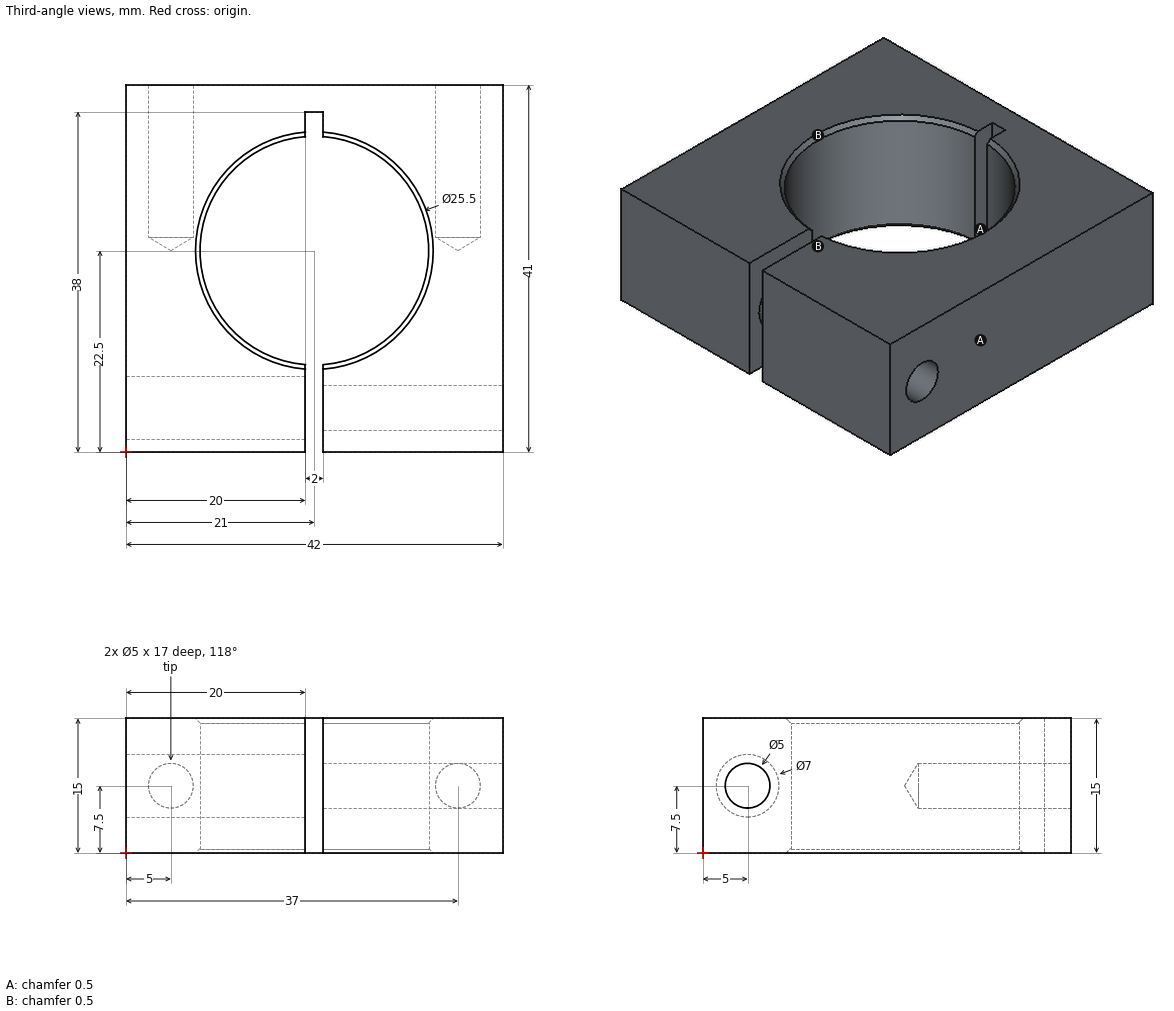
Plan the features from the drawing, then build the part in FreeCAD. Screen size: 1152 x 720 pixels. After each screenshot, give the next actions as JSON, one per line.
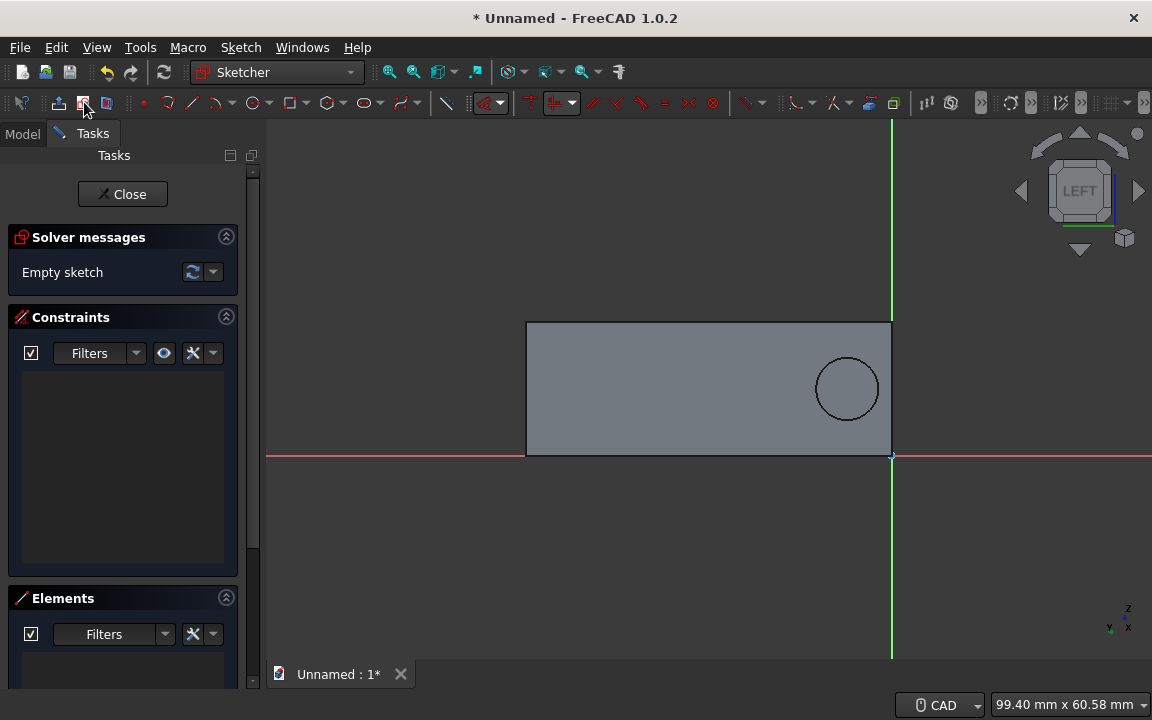
{"action": "scroll", "coordinate": [930, 419], "scroll_direction": "up", "scroll_amount": 7}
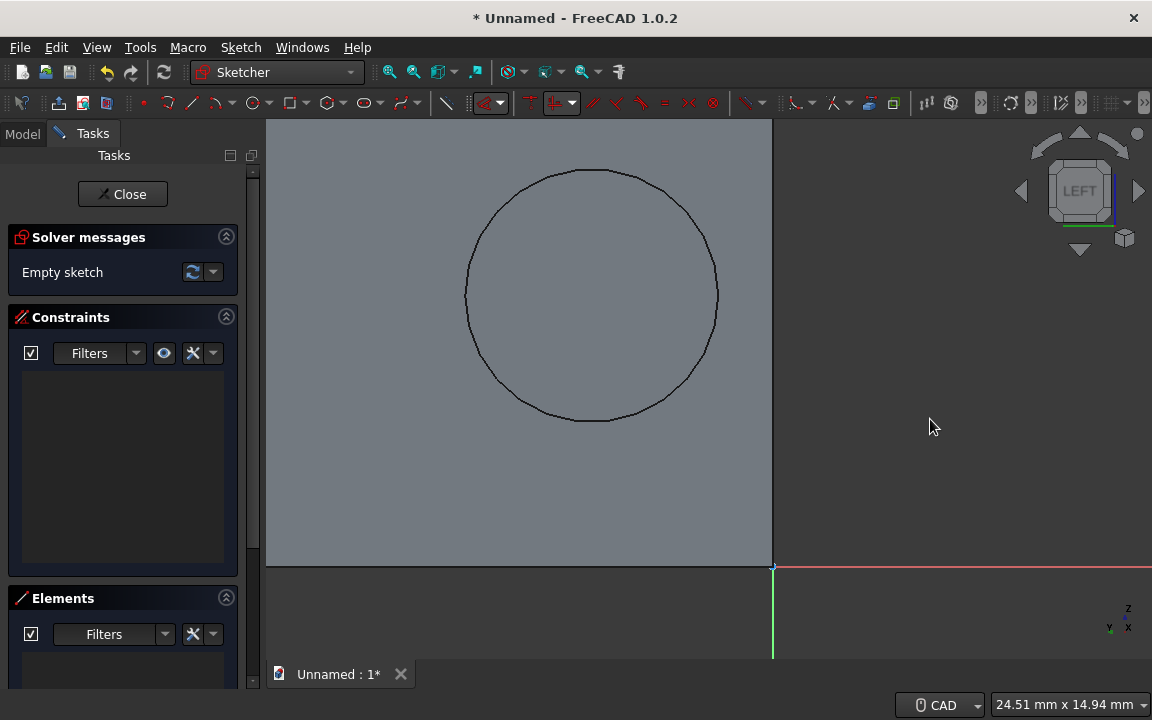
{"action": "left_click", "coordinate": [254, 104]}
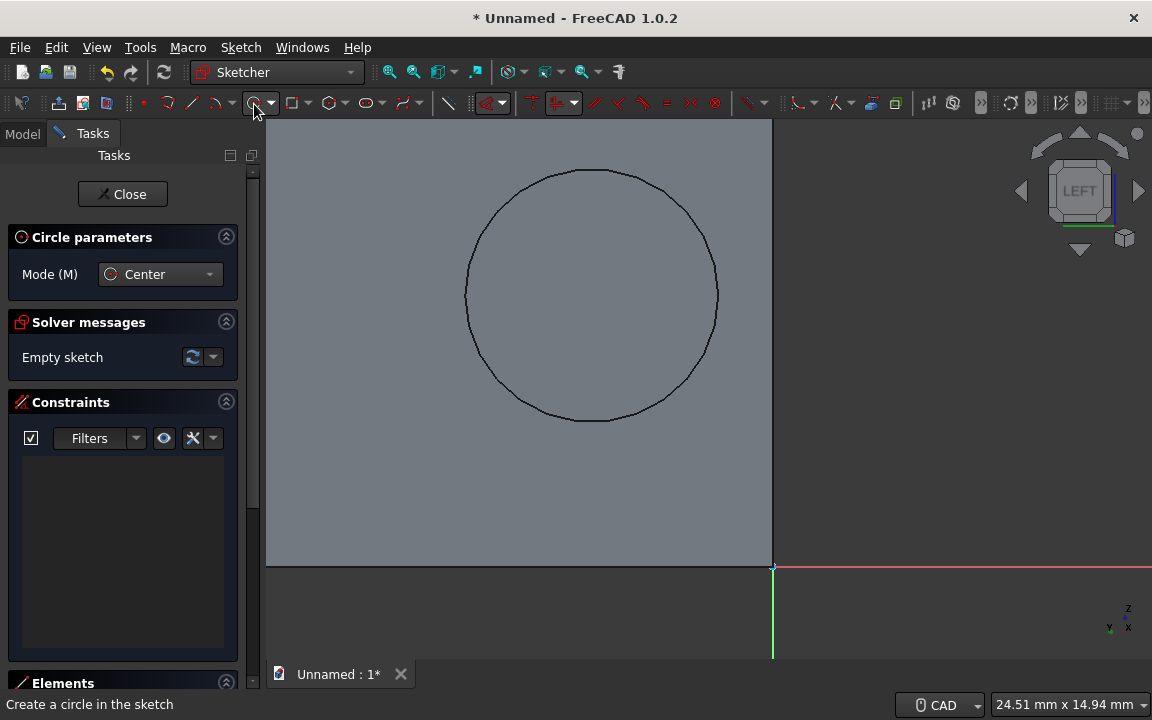
{"action": "left_click", "coordinate": [592, 296]}
{"action": "mouse_move", "coordinate": [656, 232]}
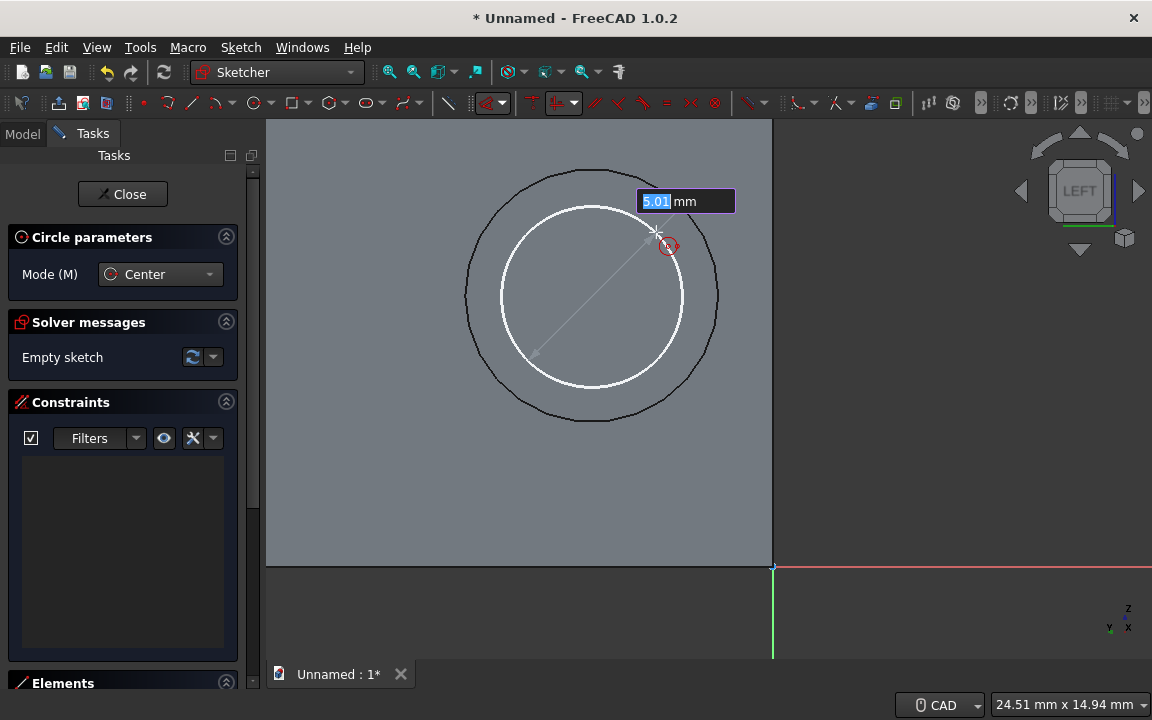
{"action": "type", "text": "5"}
{"action": "key", "text": "Return"}
{"action": "key", "text": "Escape"}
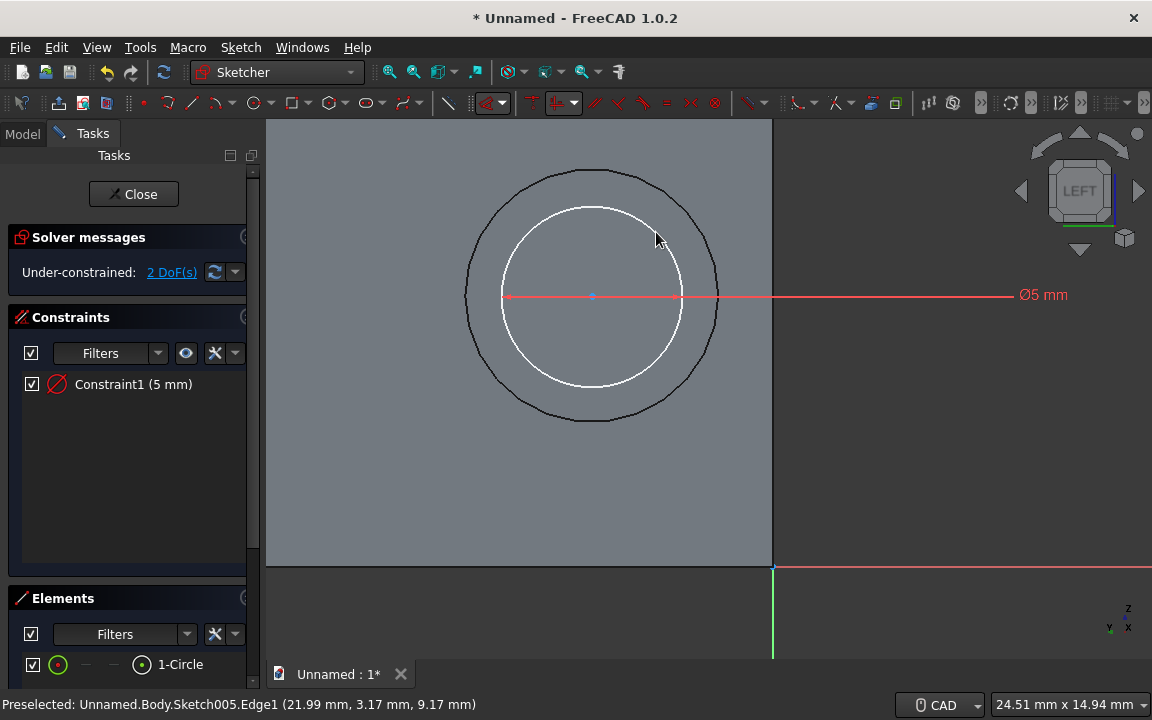
{"action": "left_click", "coordinate": [592, 297]}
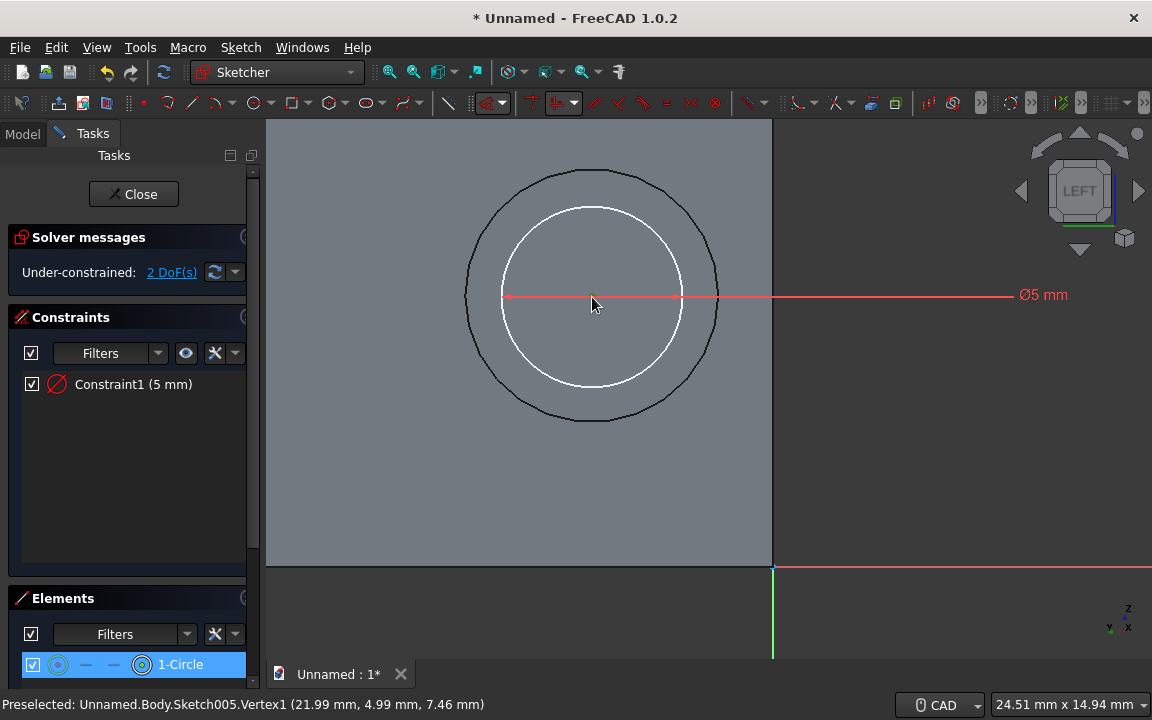
{"action": "left_click", "coordinate": [504, 104]}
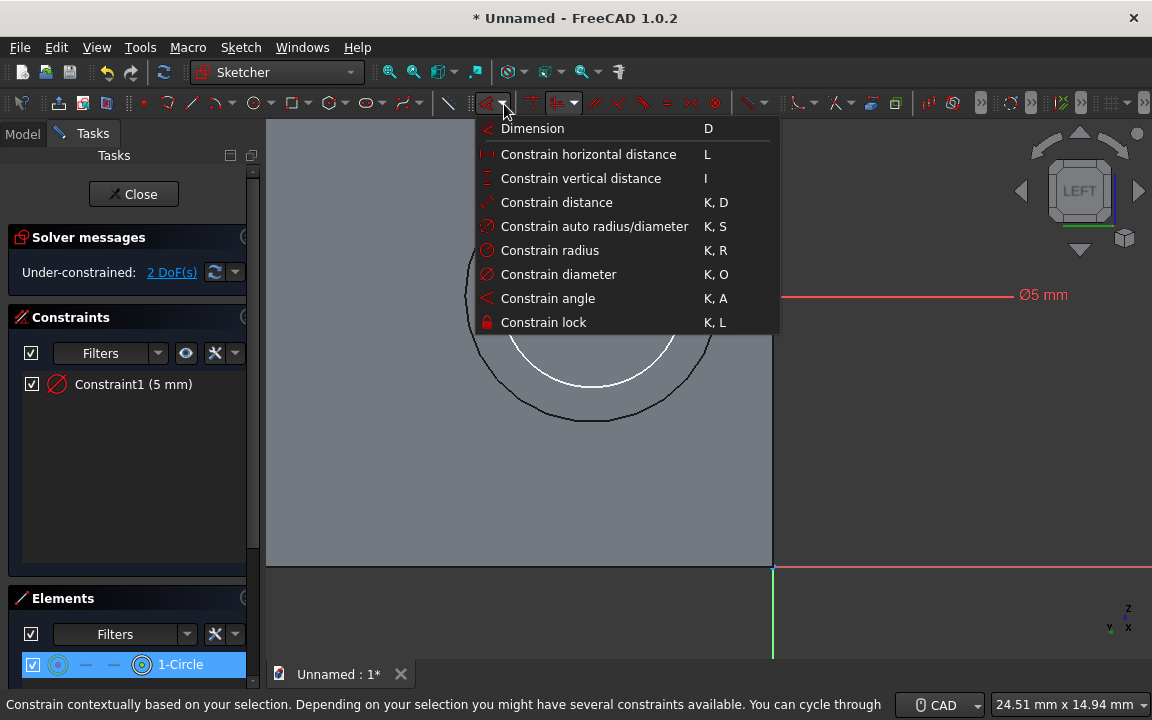
{"action": "left_click", "coordinate": [628, 154]}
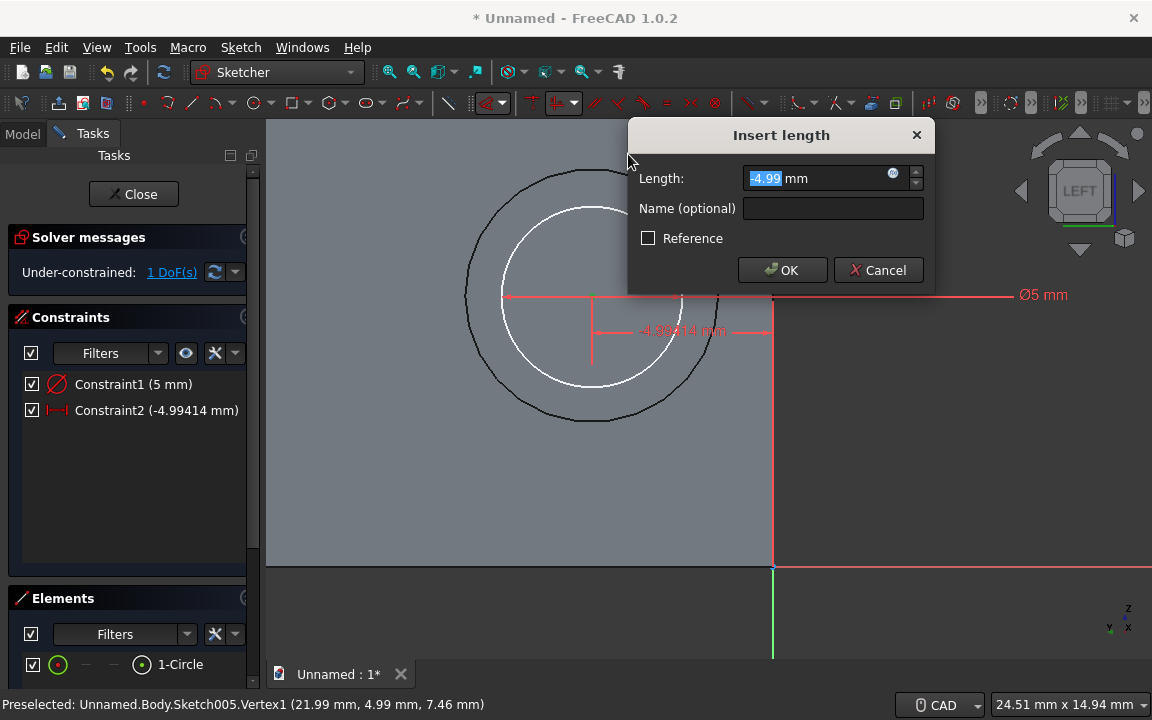
{"action": "type", "text": "-5"}
{"action": "key", "text": "Return"}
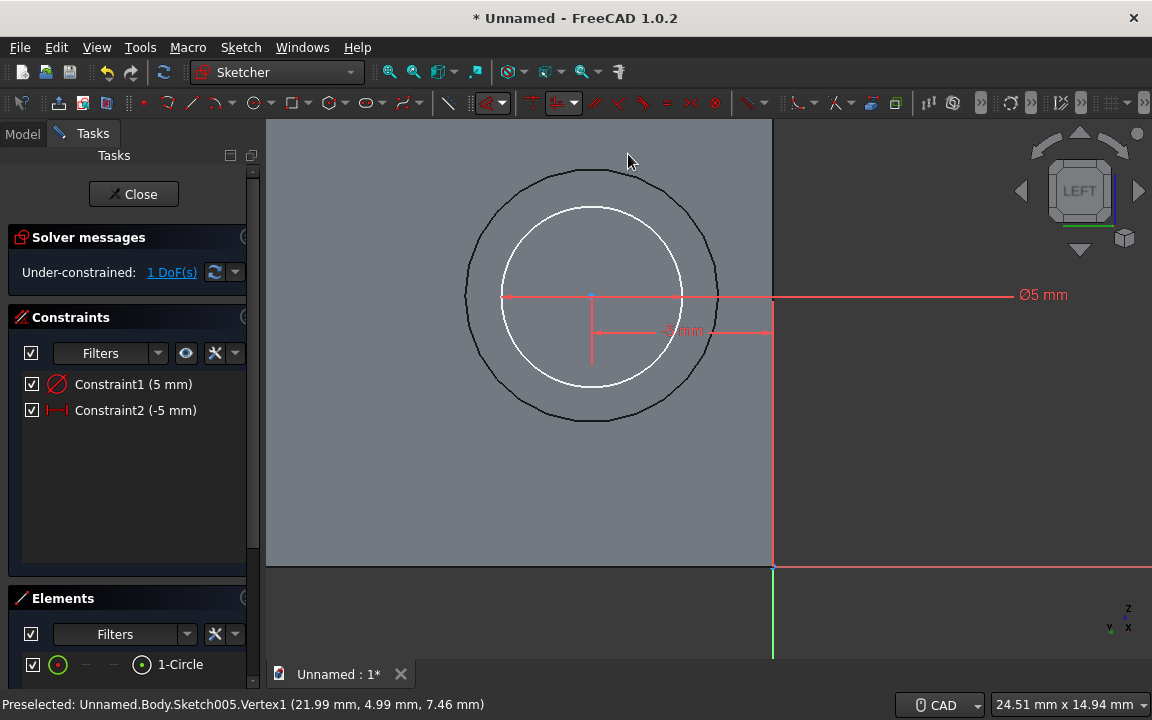
{"action": "left_click", "coordinate": [592, 297]}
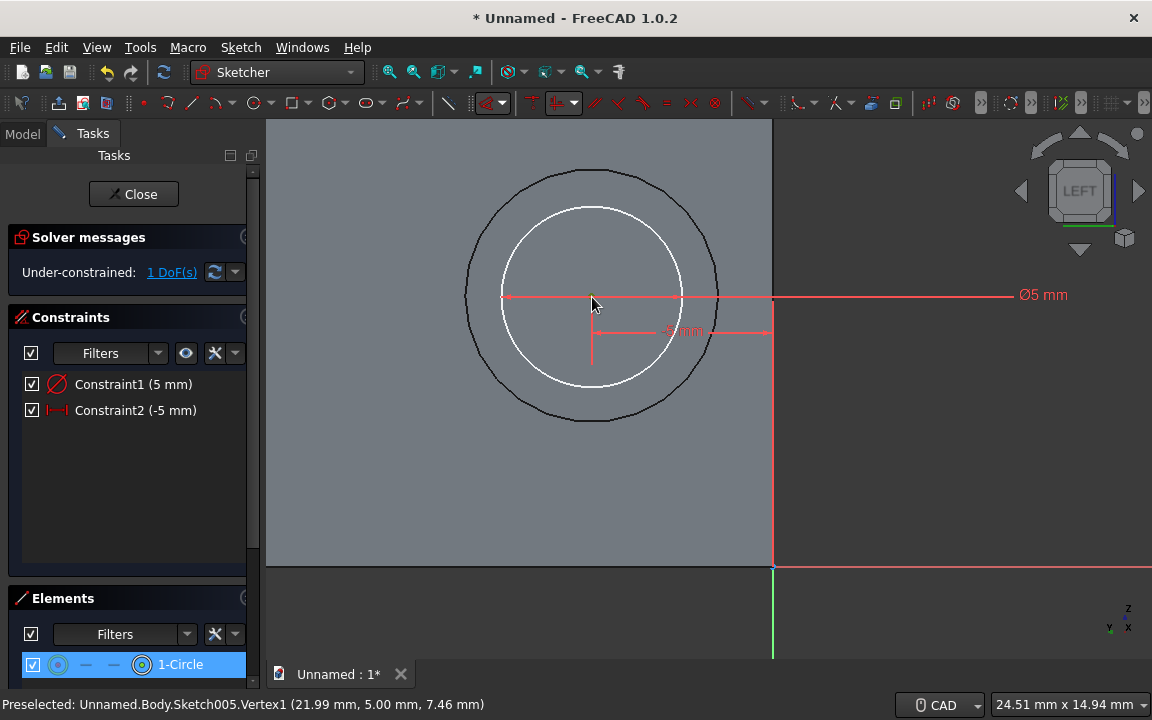
{"action": "left_click", "coordinate": [504, 104]}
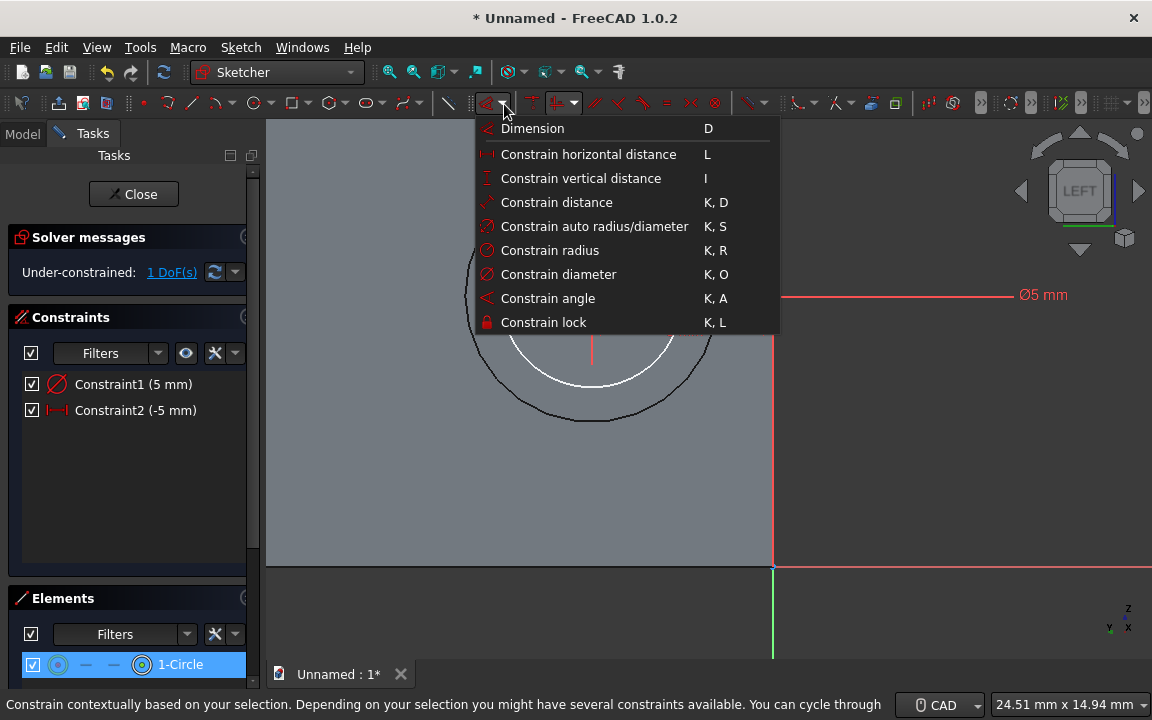
{"action": "left_click", "coordinate": [628, 178]}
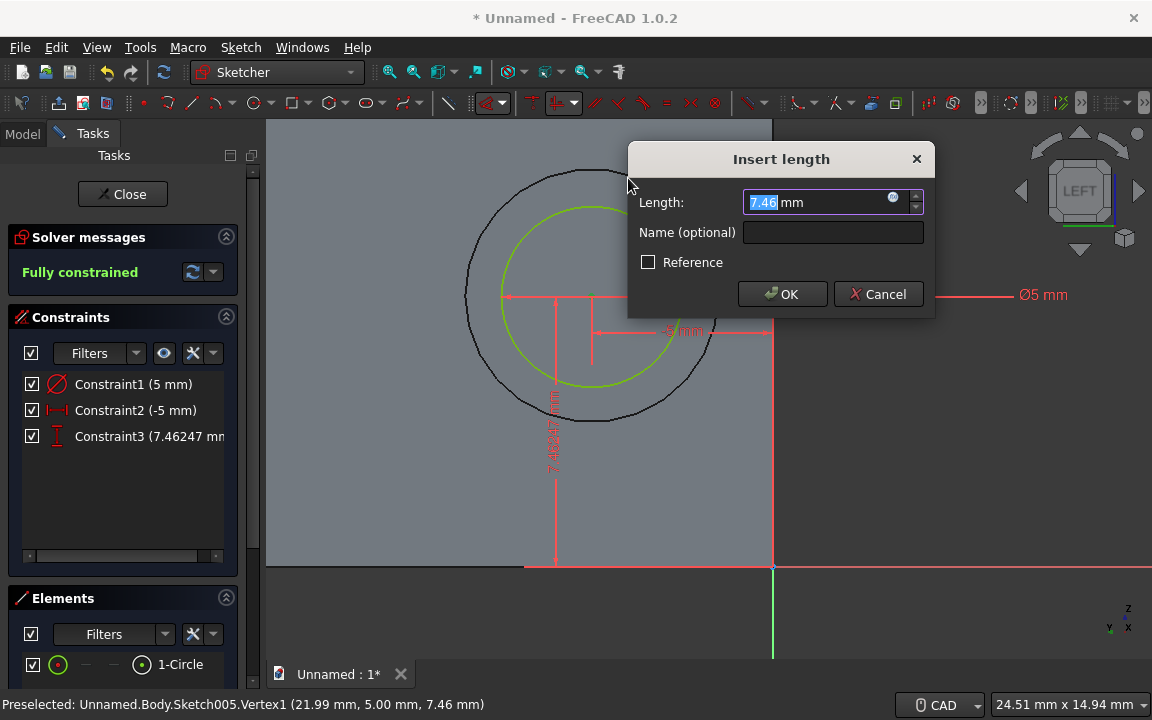
{"action": "type", "text": "7.5"}
{"action": "key", "text": "Return"}